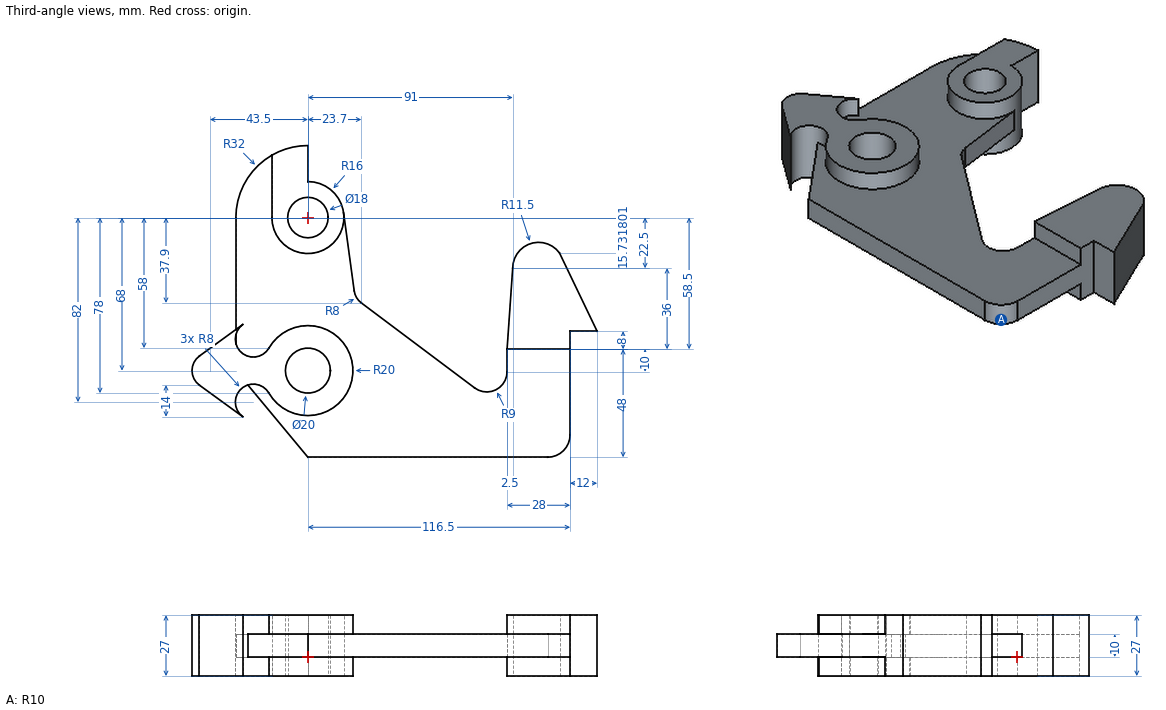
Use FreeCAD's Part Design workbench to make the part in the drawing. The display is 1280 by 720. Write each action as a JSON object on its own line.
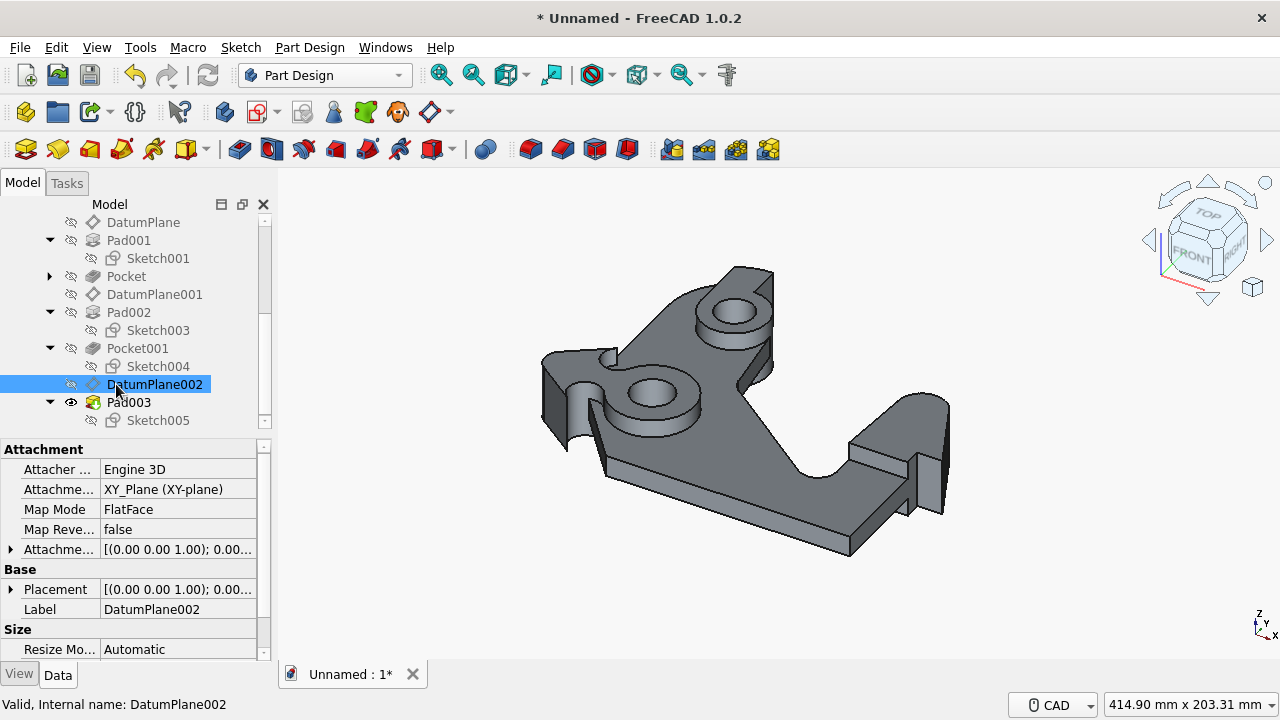
{"action": "left_click", "coordinate": [850, 545]}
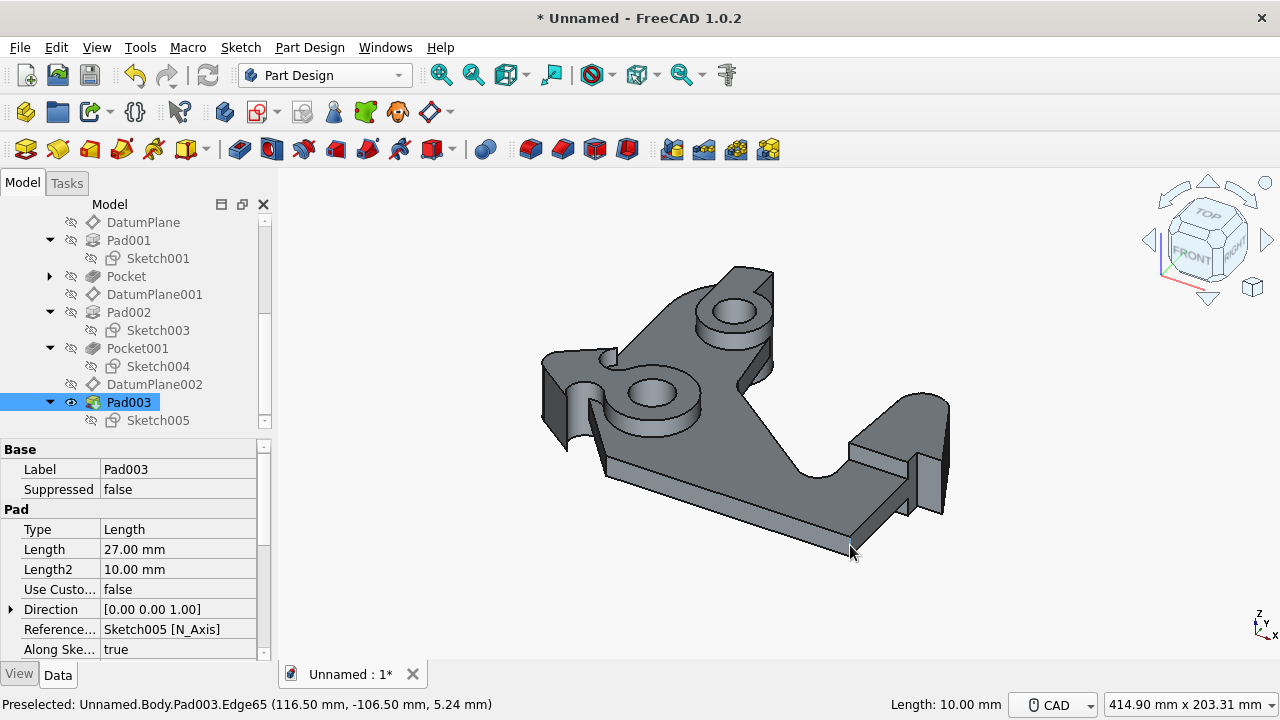
{"action": "left_click", "coordinate": [532, 150]}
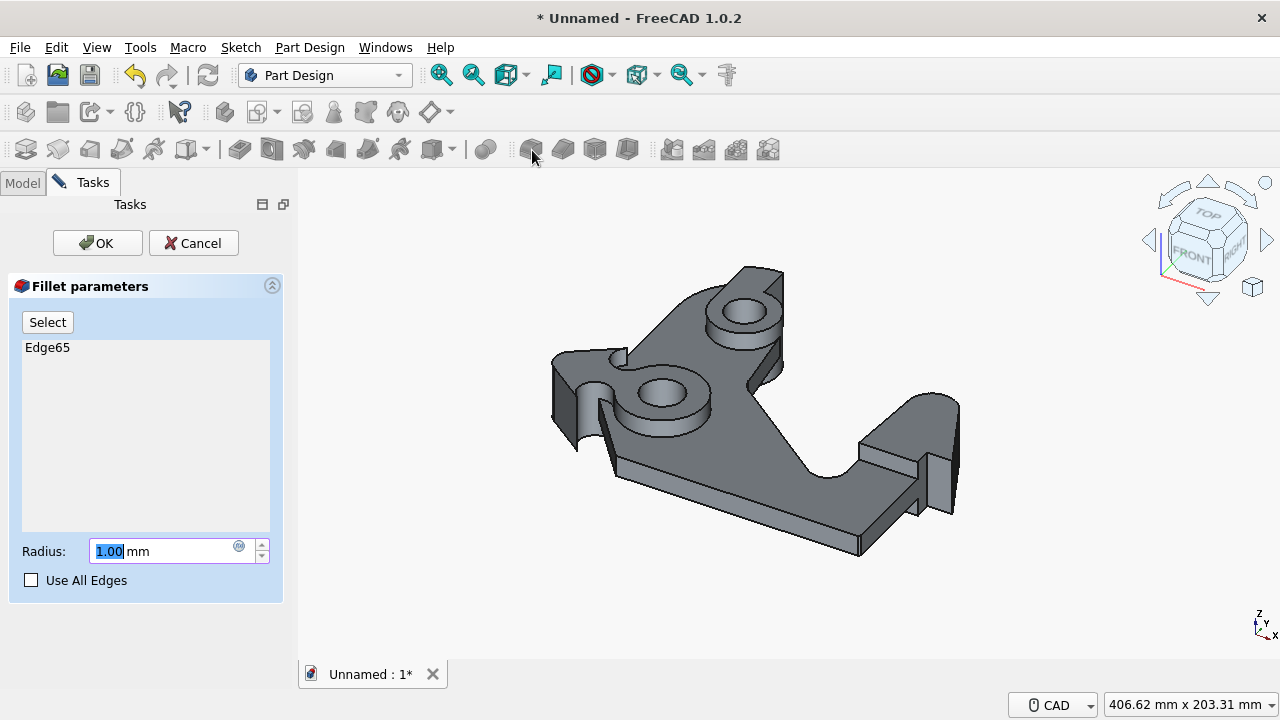
{"action": "type", "text": "10"}
{"action": "key", "text": "Tab"}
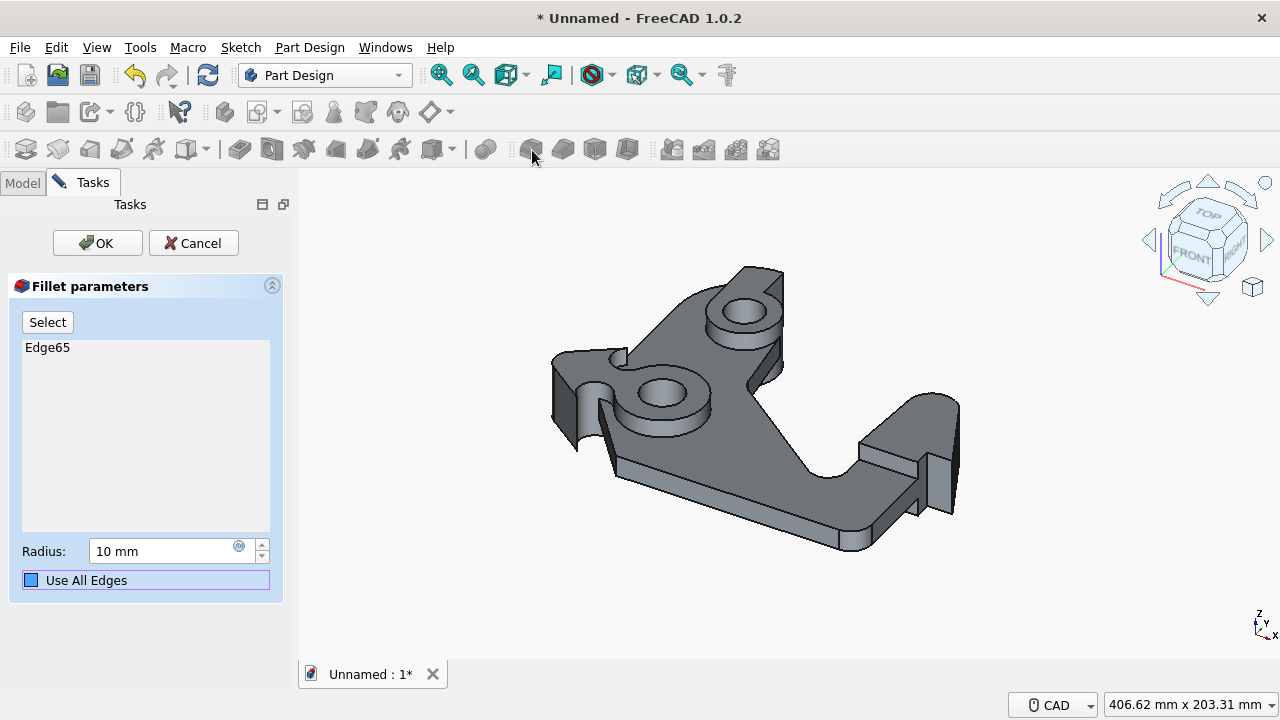
{"action": "left_click", "coordinate": [98, 243]}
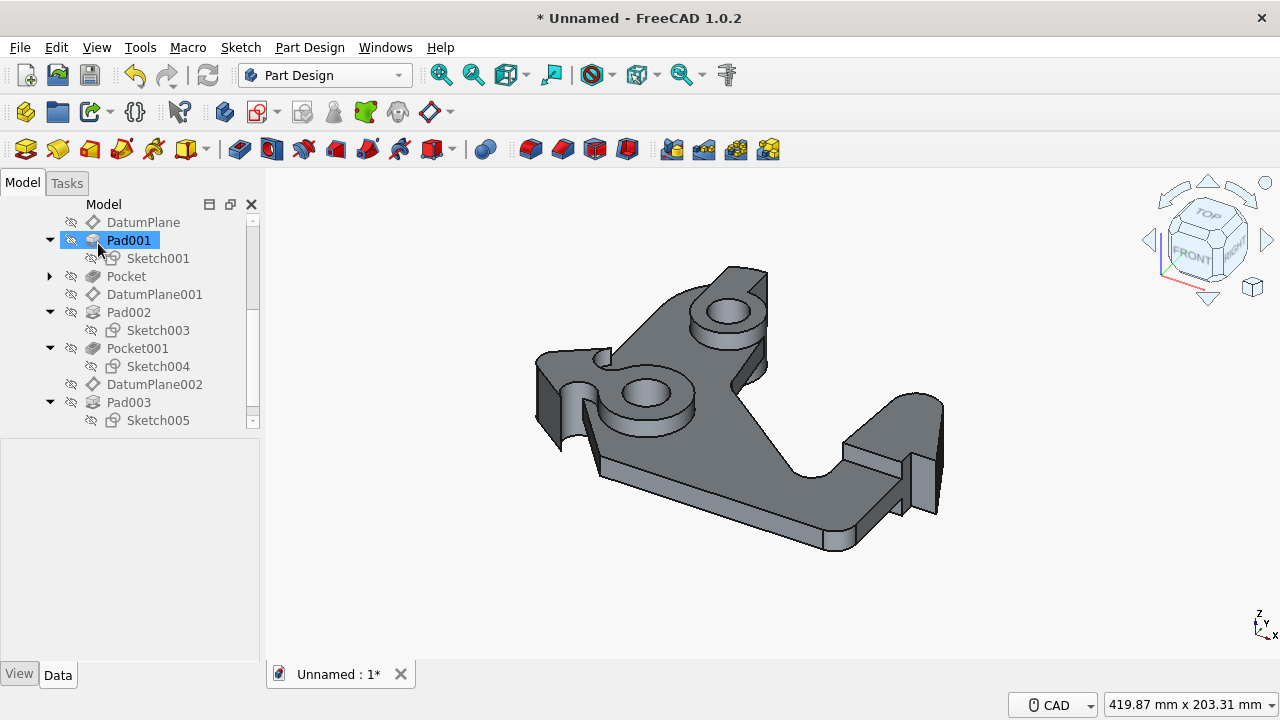
{"action": "key", "text": "0"}